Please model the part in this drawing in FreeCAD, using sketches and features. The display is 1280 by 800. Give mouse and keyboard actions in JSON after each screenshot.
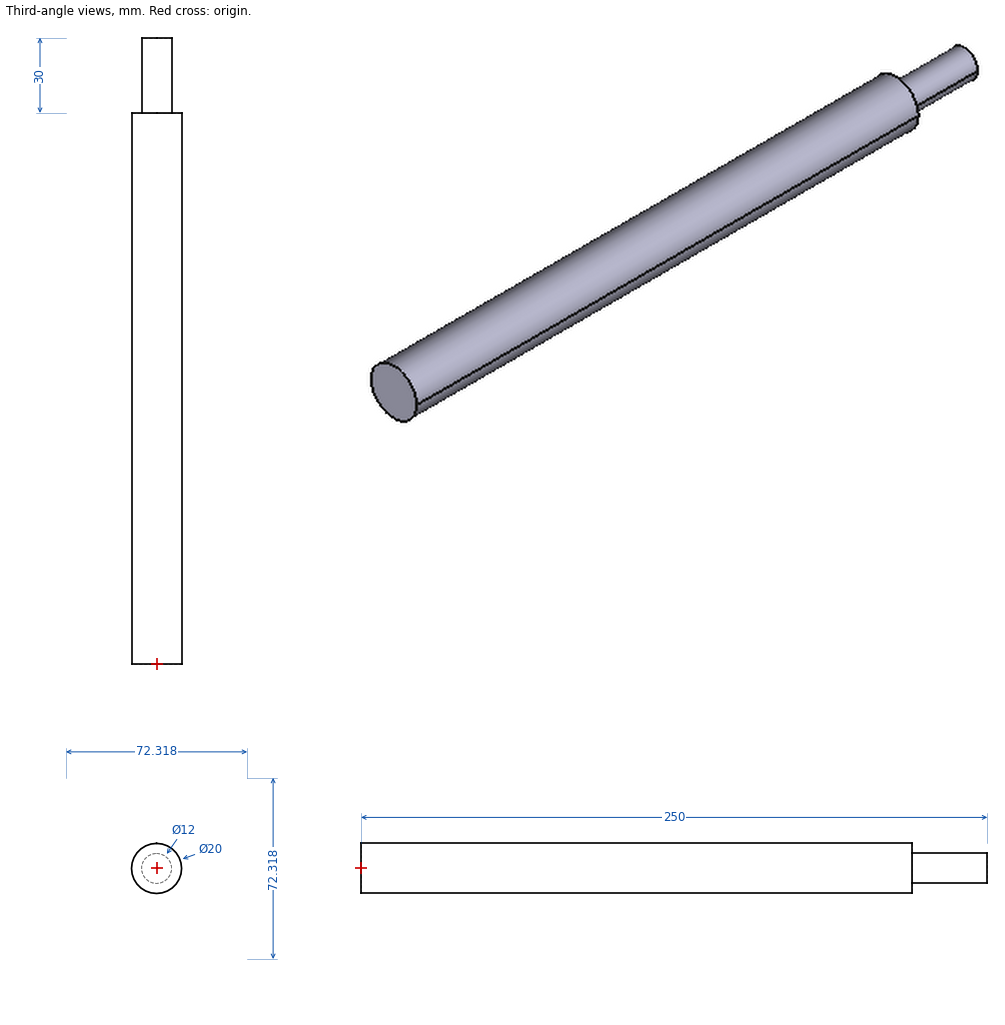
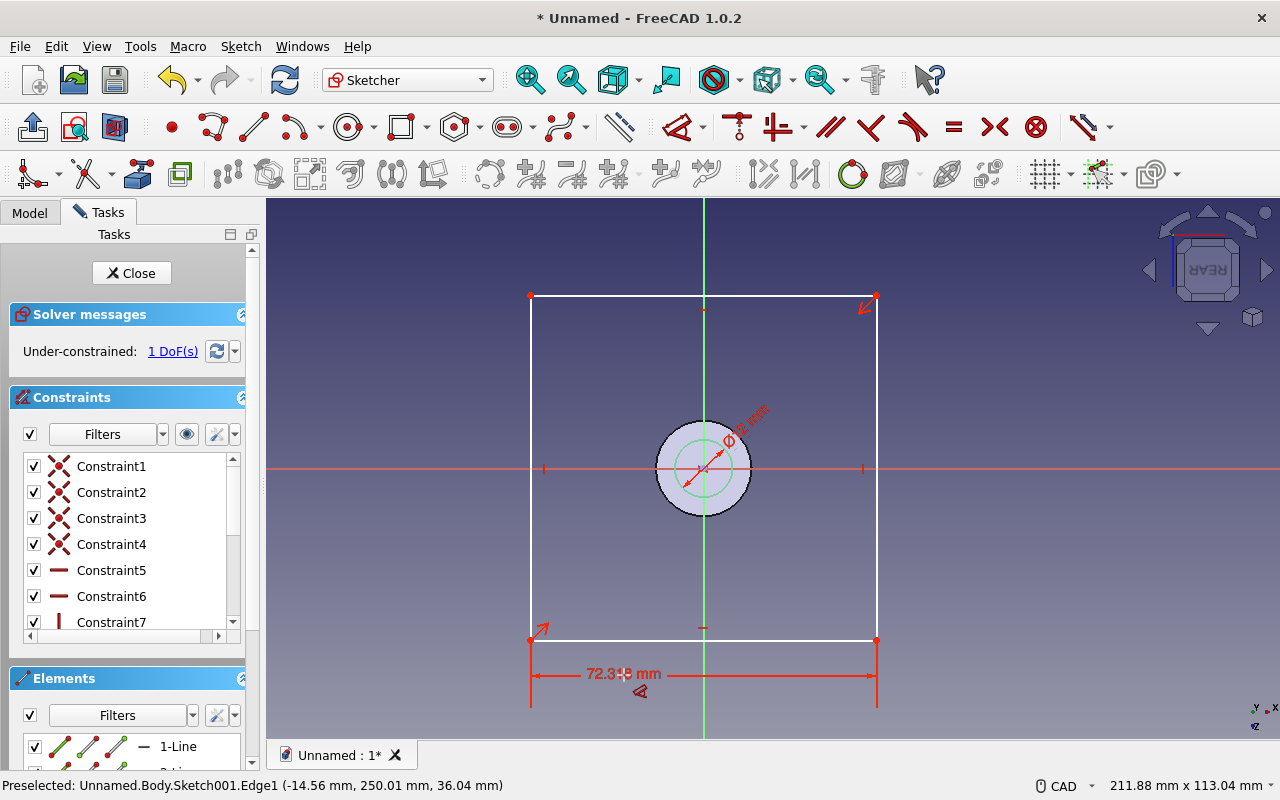
{"action": "left_click", "coordinate": [877, 537]}
{"action": "left_click", "coordinate": [911, 389]}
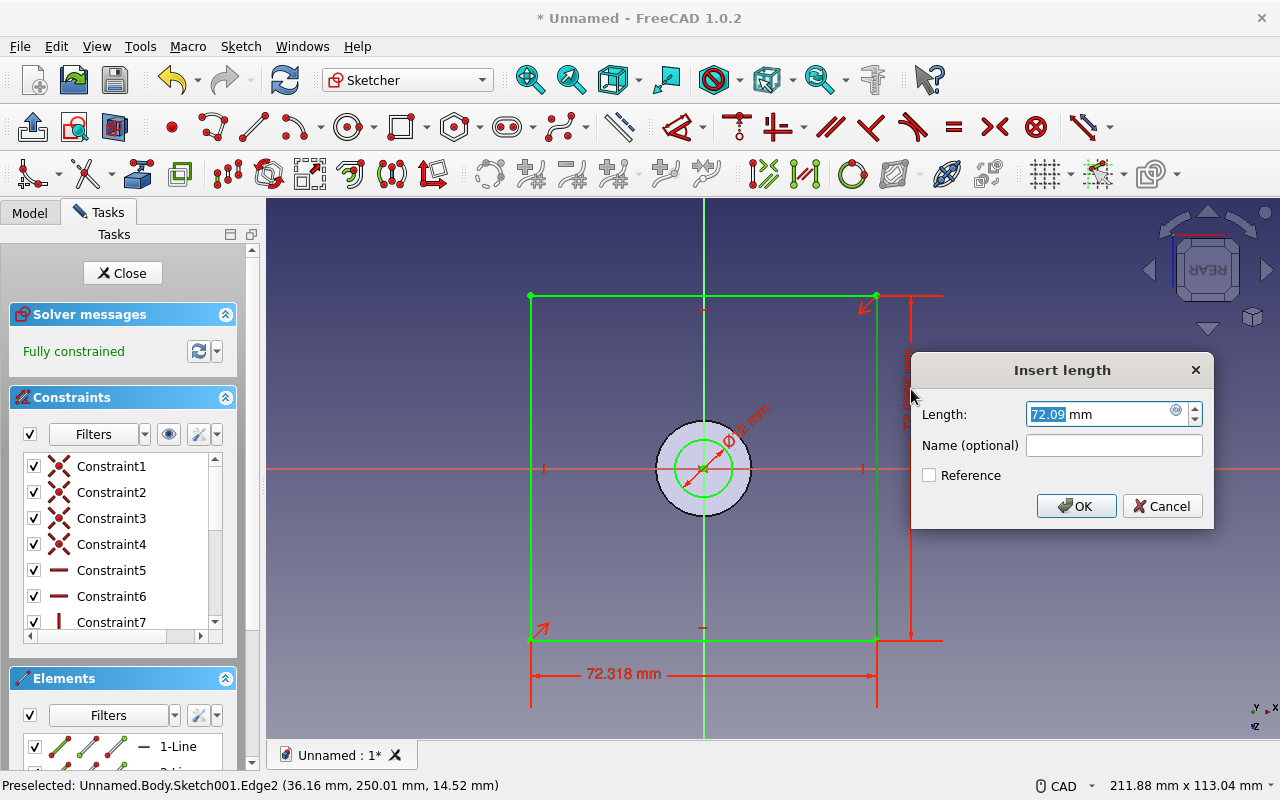
{"action": "type", "text": "72.318"}
{"action": "key", "text": "Return"}
{"action": "key", "text": "Escape"}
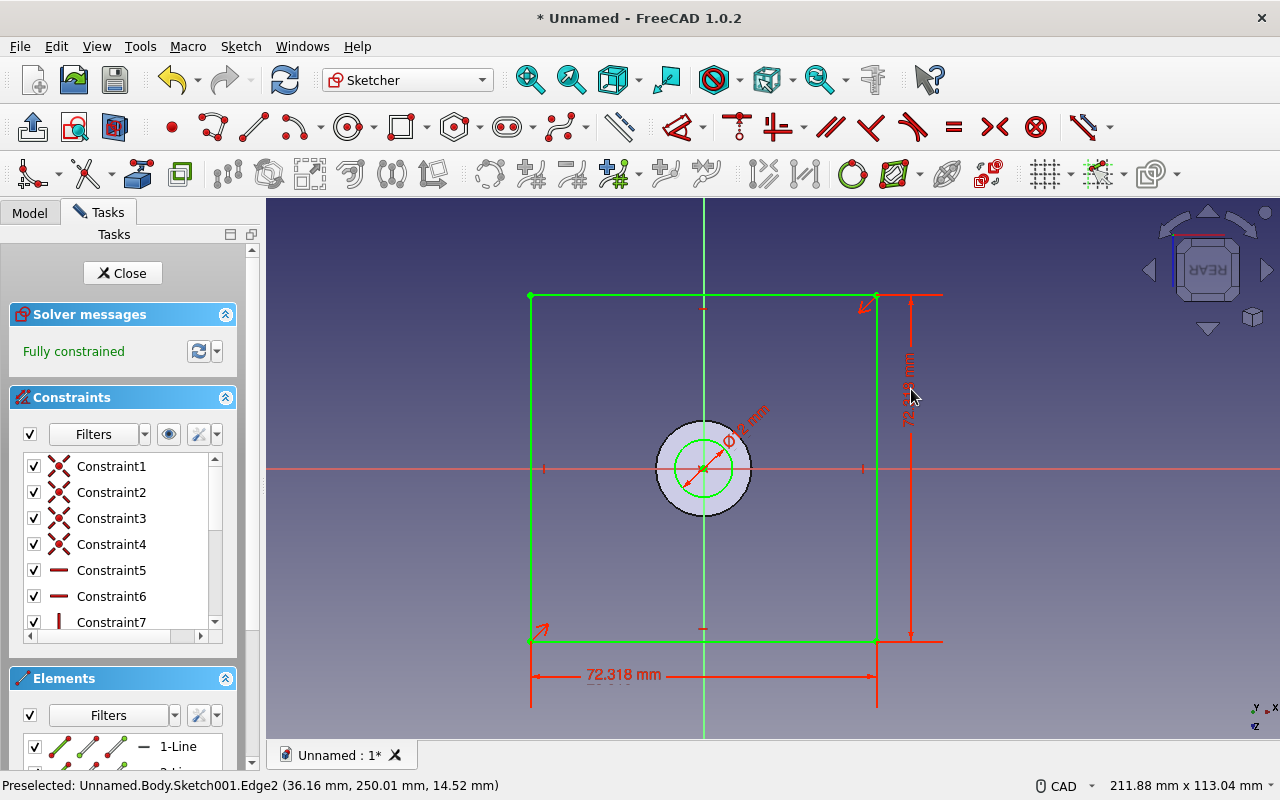
{"action": "left_click", "coordinate": [123, 273]}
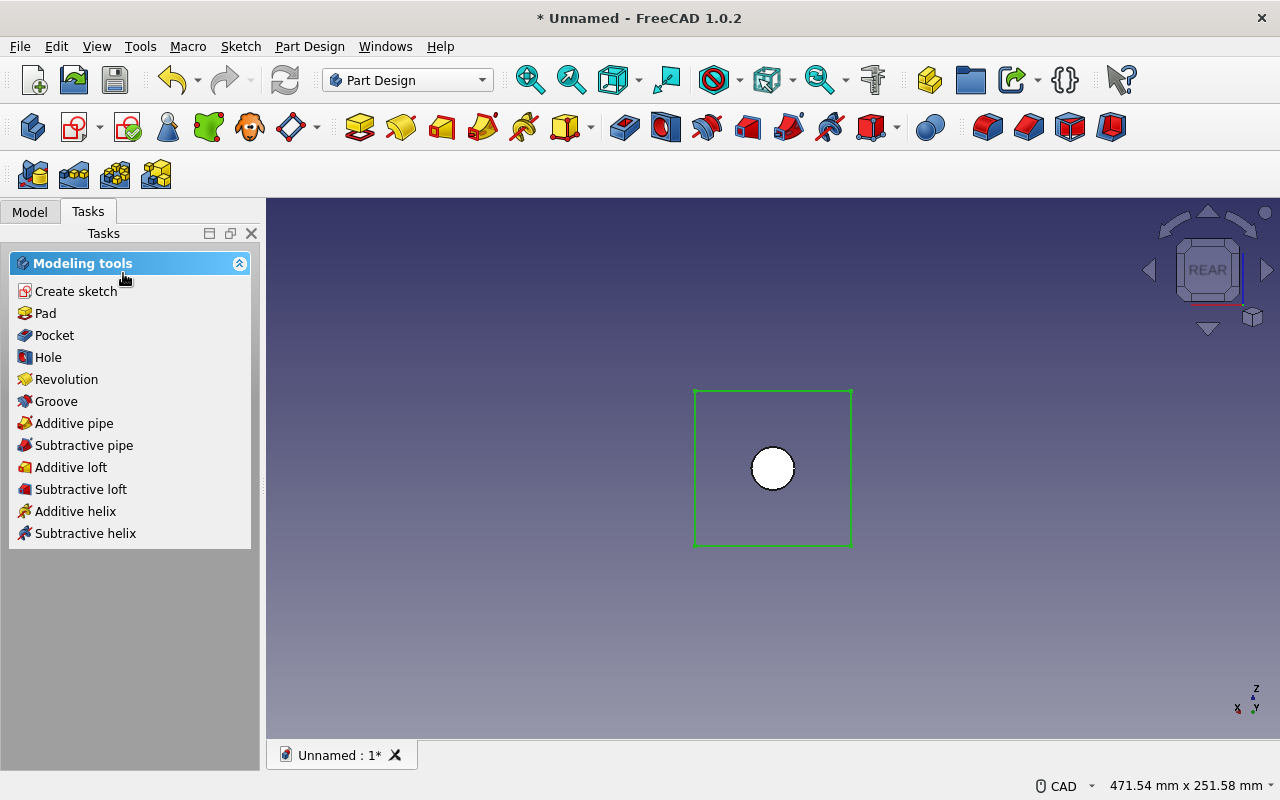
{"action": "left_click", "coordinate": [625, 128]}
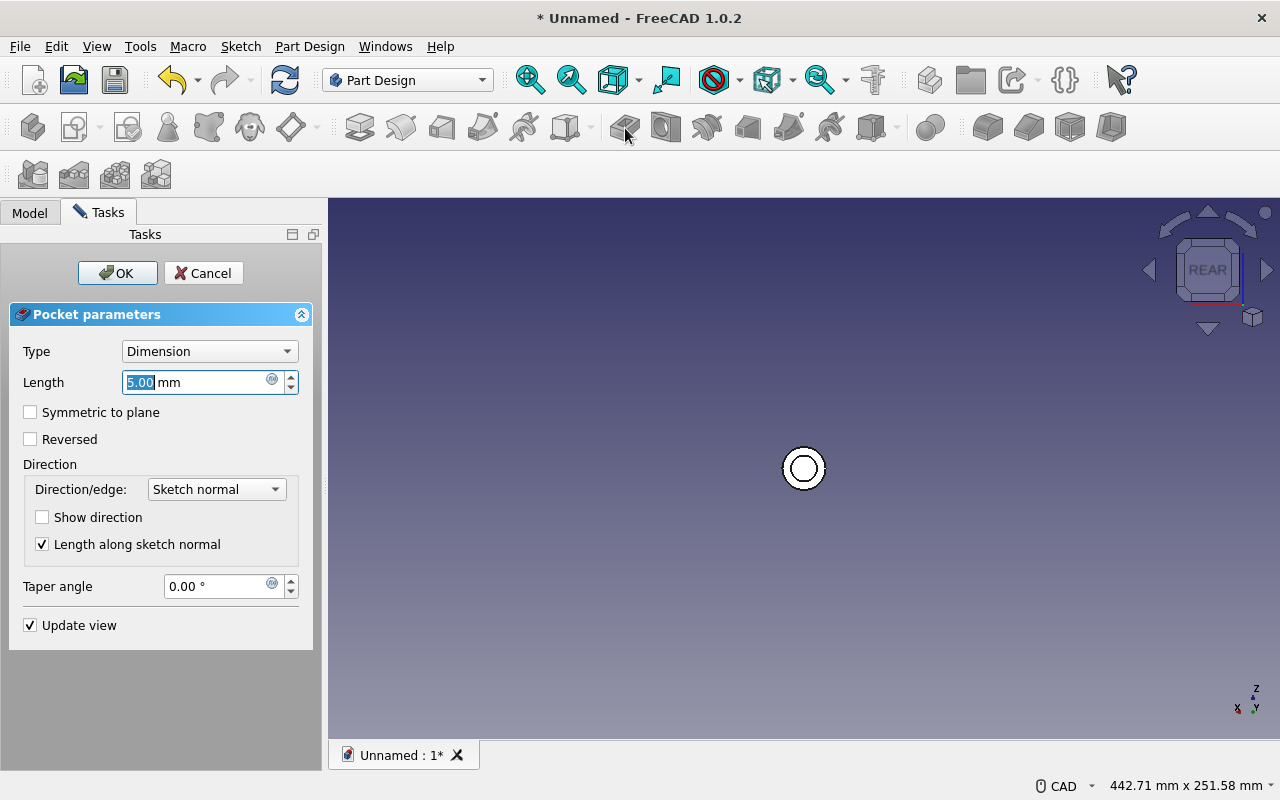
{"action": "type", "text": "30"}
{"action": "key", "text": "Tab"}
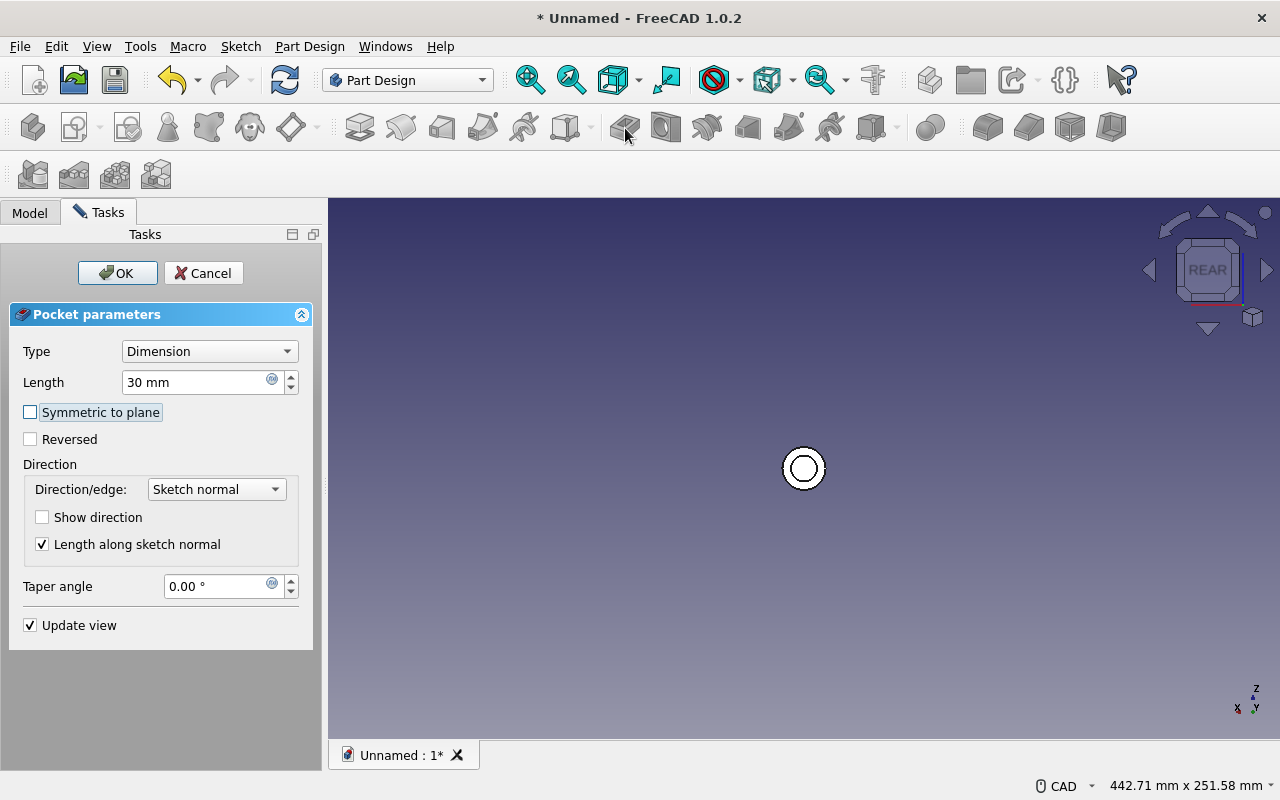
{"action": "left_click", "coordinate": [118, 273]}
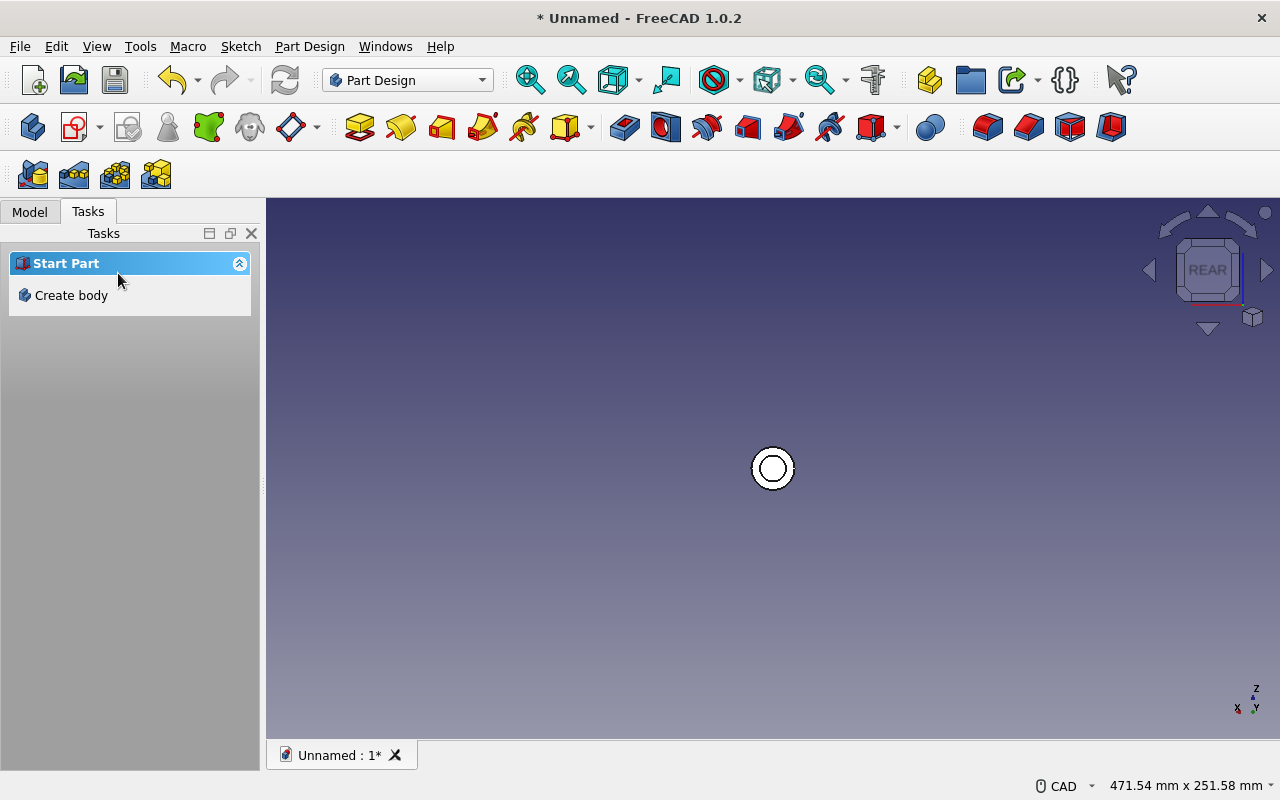
{"action": "key", "text": "0"}